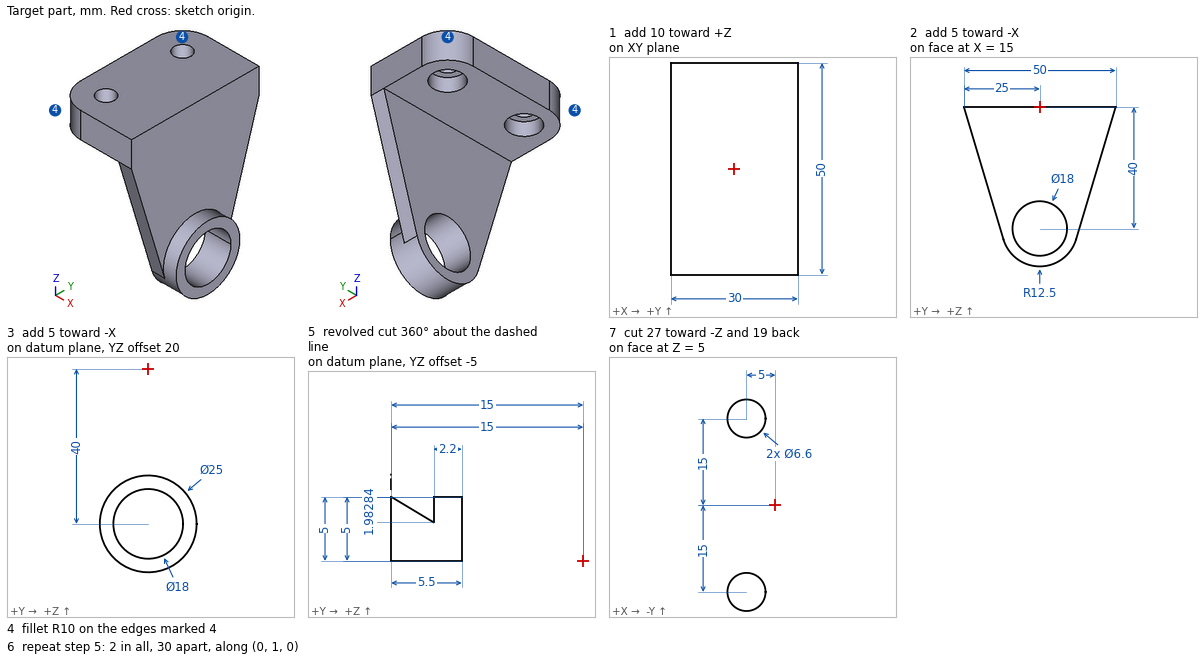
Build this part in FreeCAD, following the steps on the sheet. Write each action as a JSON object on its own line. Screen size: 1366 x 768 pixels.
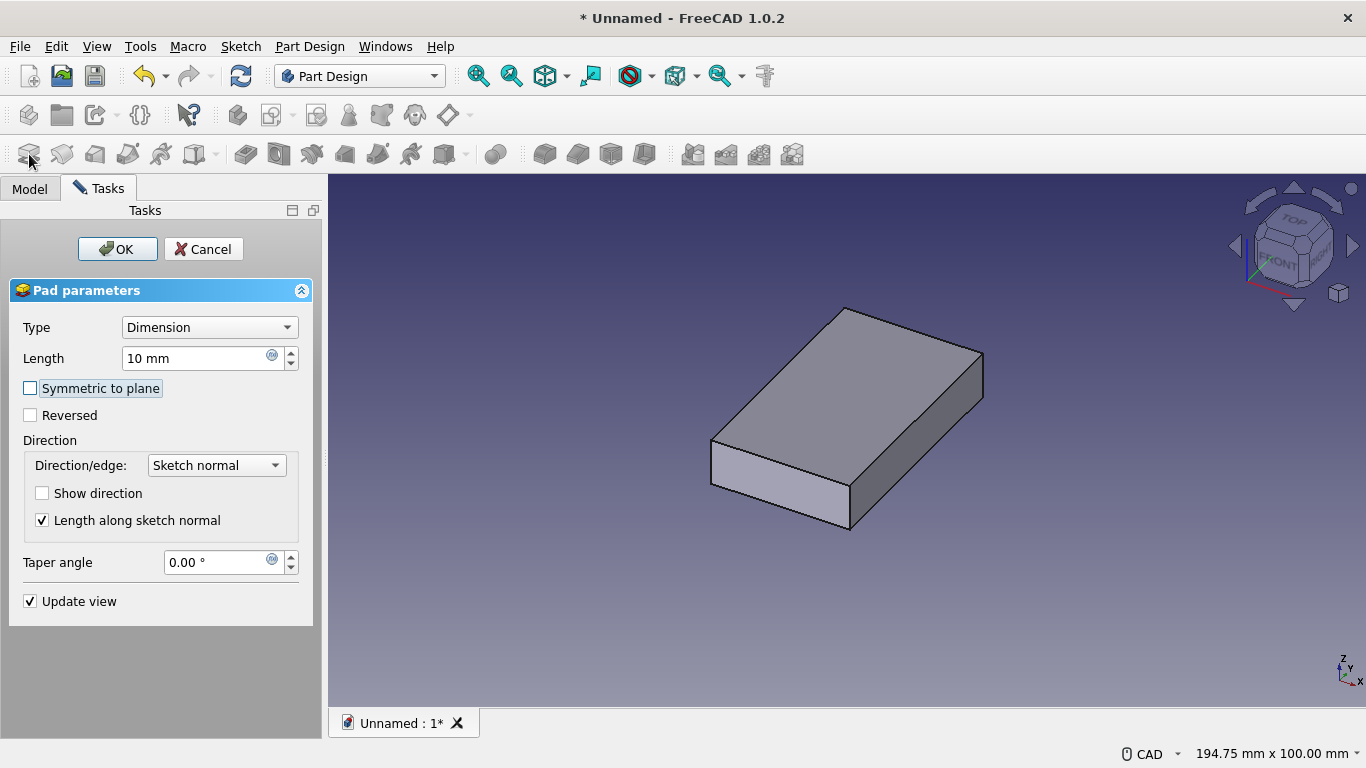
{"action": "left_click", "coordinate": [118, 249]}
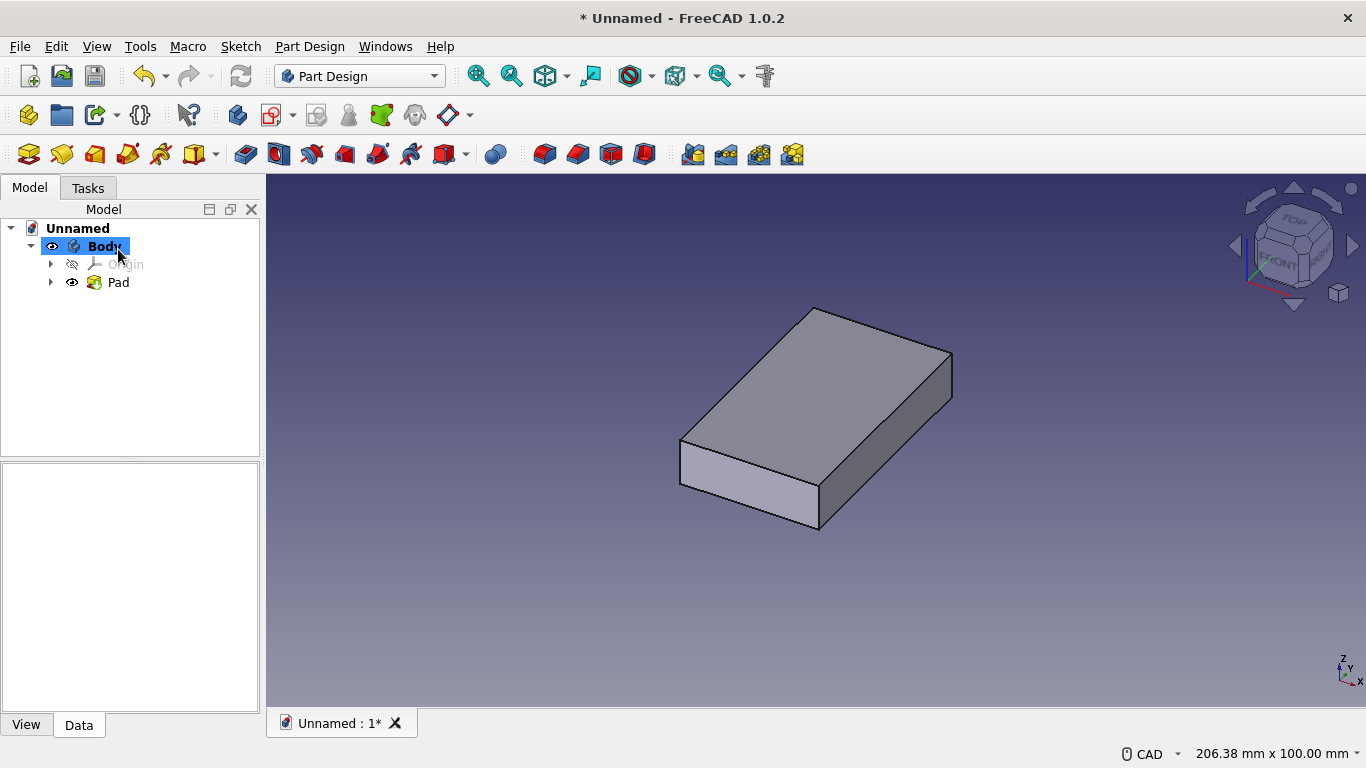
{"action": "key", "text": "v f"}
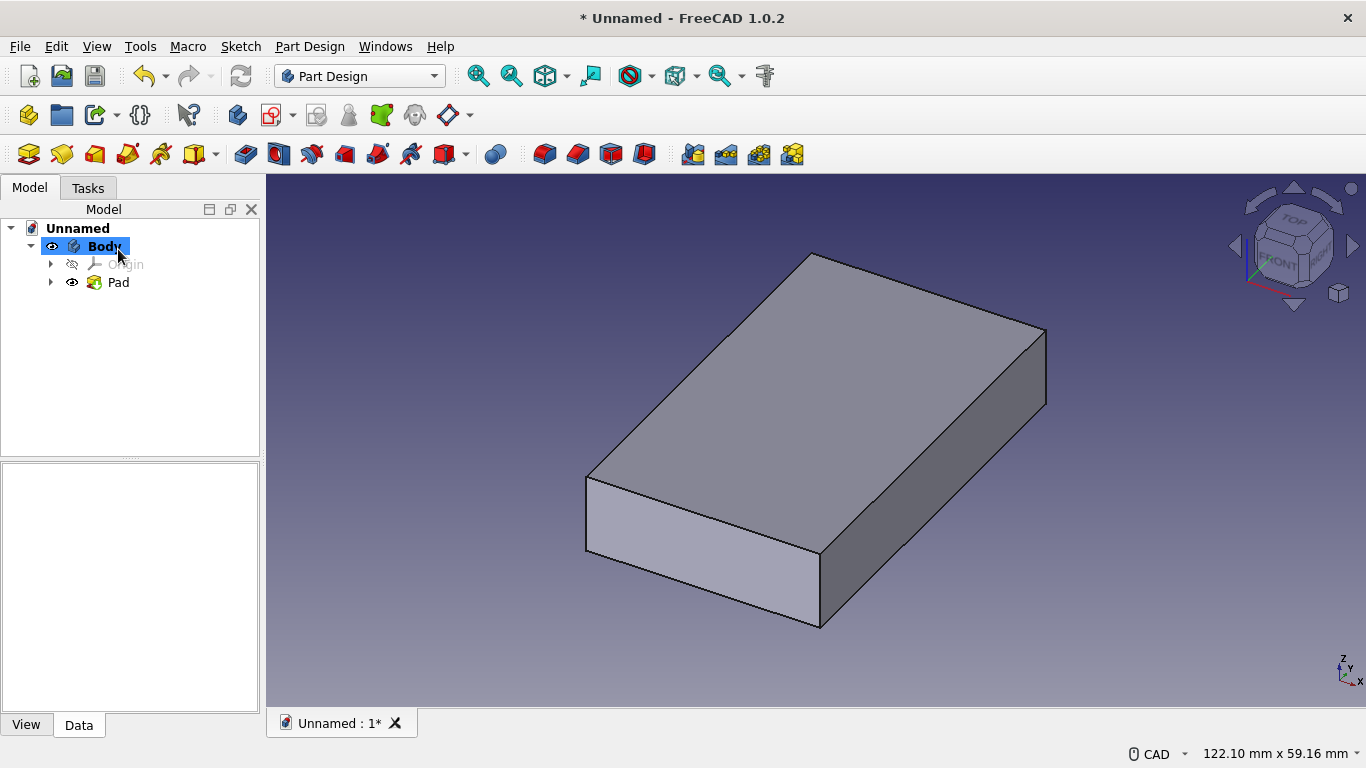
{"action": "left_click", "coordinate": [997, 414]}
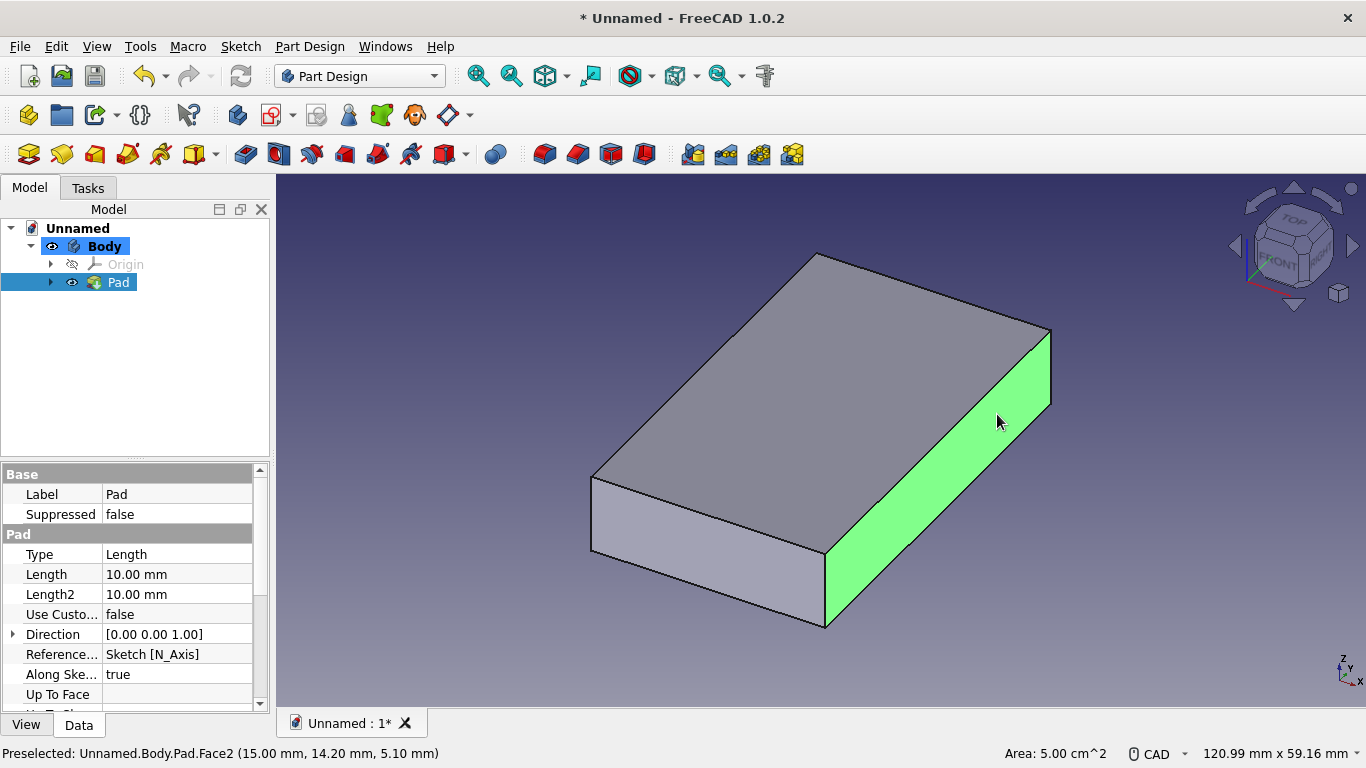
{"action": "left_click", "coordinate": [270, 116]}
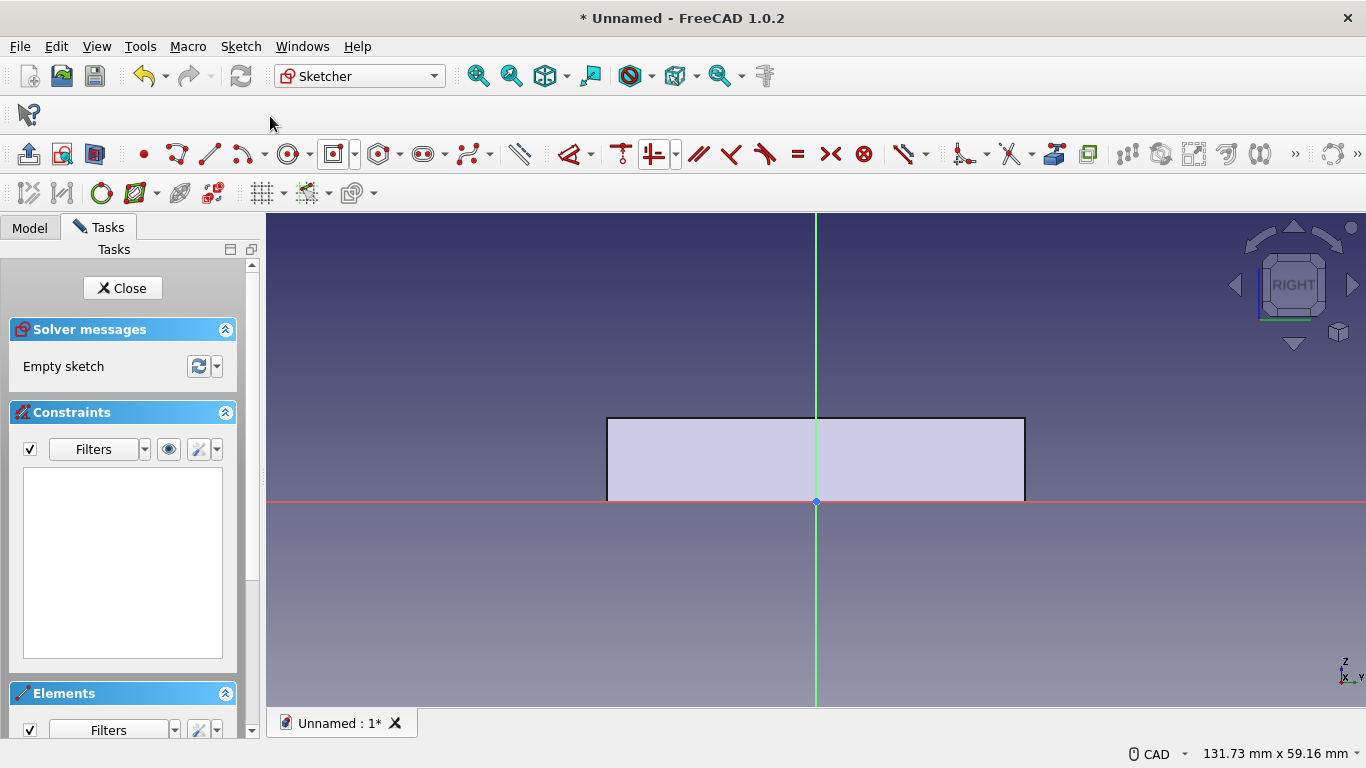
{"action": "scroll", "coordinate": [664, 241], "scroll_direction": "down", "scroll_amount": 3}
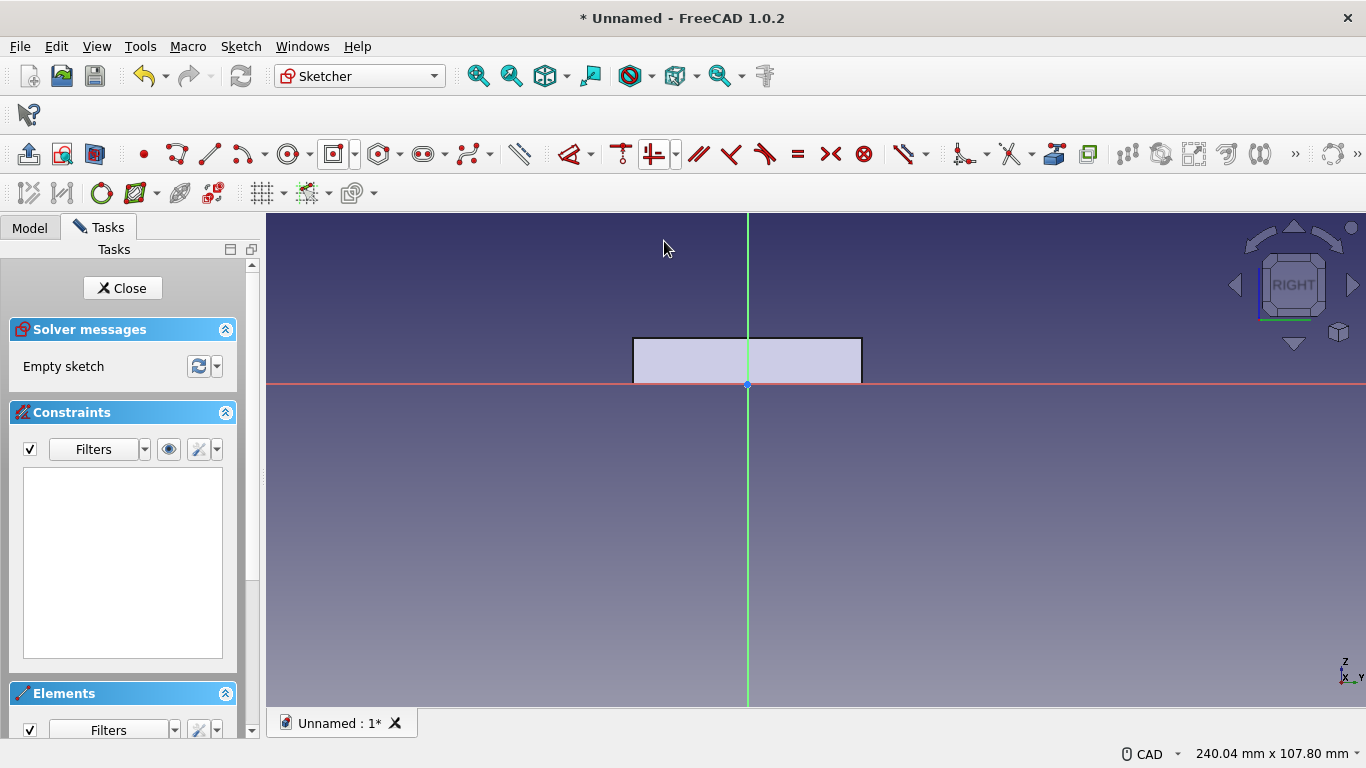
{"action": "left_click", "coordinate": [177, 154]}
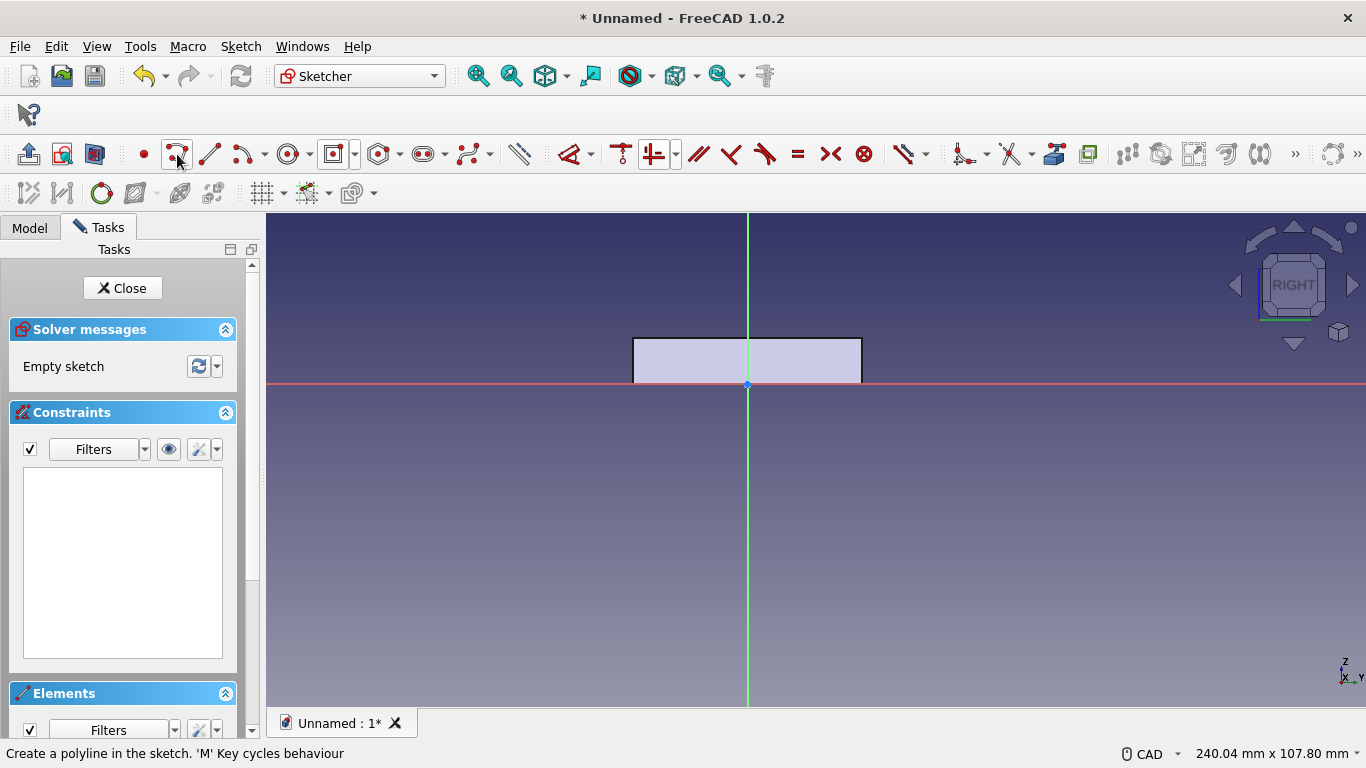
{"action": "left_click", "coordinate": [693, 584]}
{"action": "left_click", "coordinate": [633, 384]}
{"action": "left_click", "coordinate": [862, 393]}
{"action": "left_click", "coordinate": [802, 584]}
{"action": "right_click", "coordinate": [802, 584]}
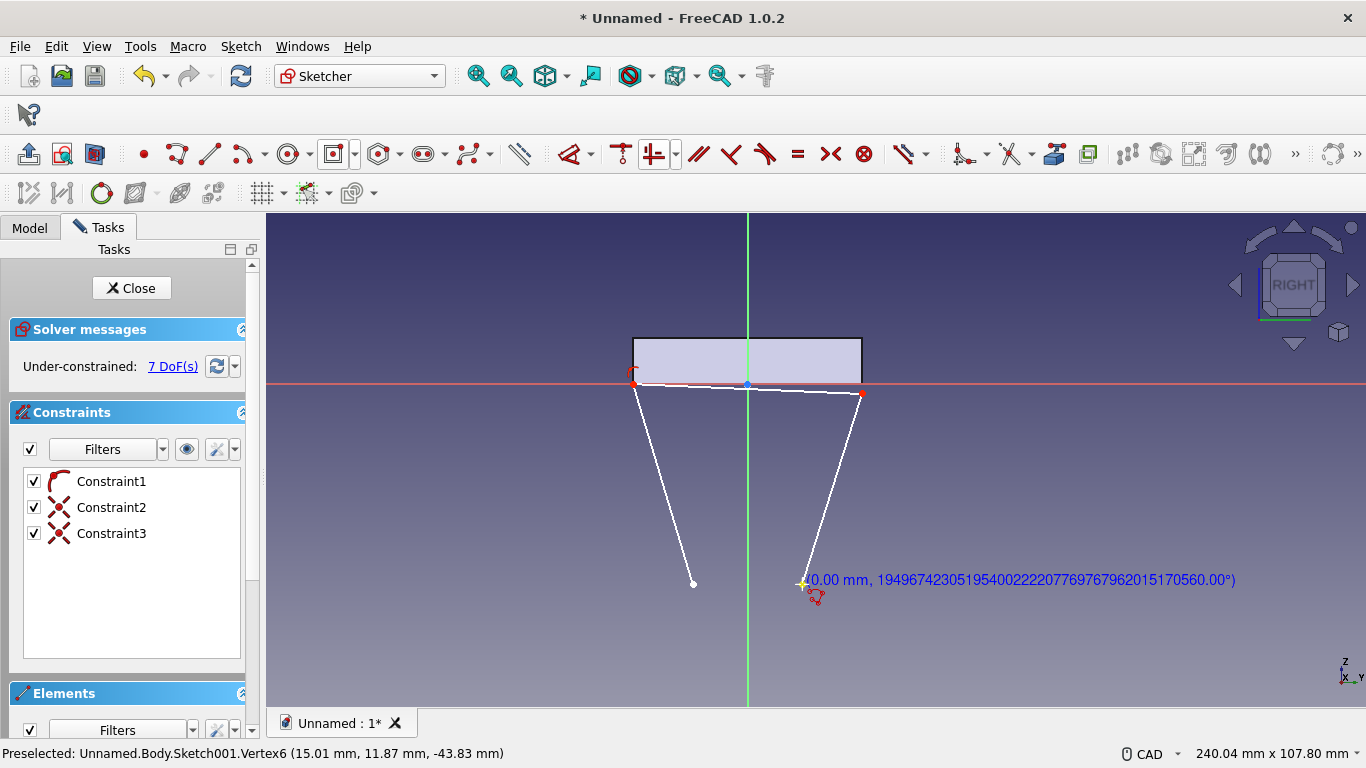
{"action": "key", "text": "g 3 a"}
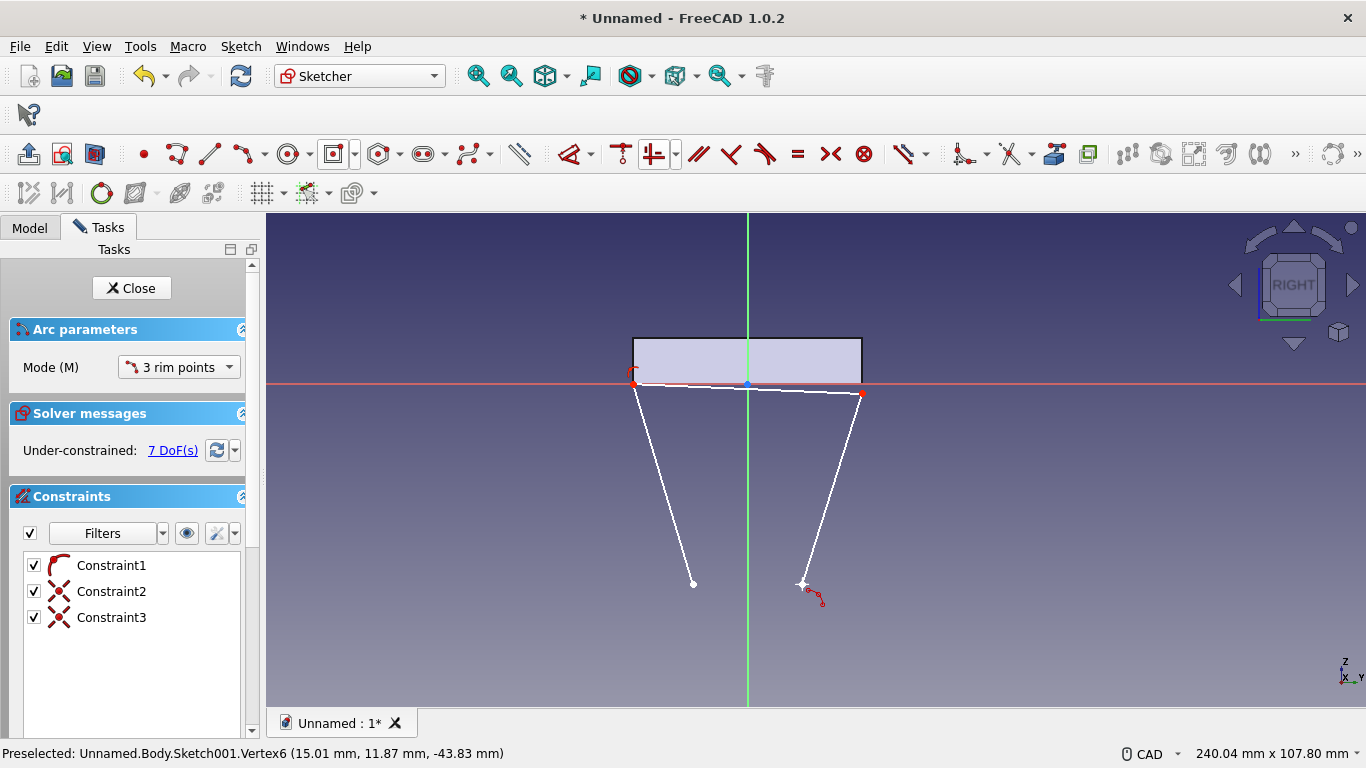
{"action": "left_click", "coordinate": [802, 585]}
{"action": "left_click", "coordinate": [693, 585]}
{"action": "left_click", "coordinate": [733, 623]}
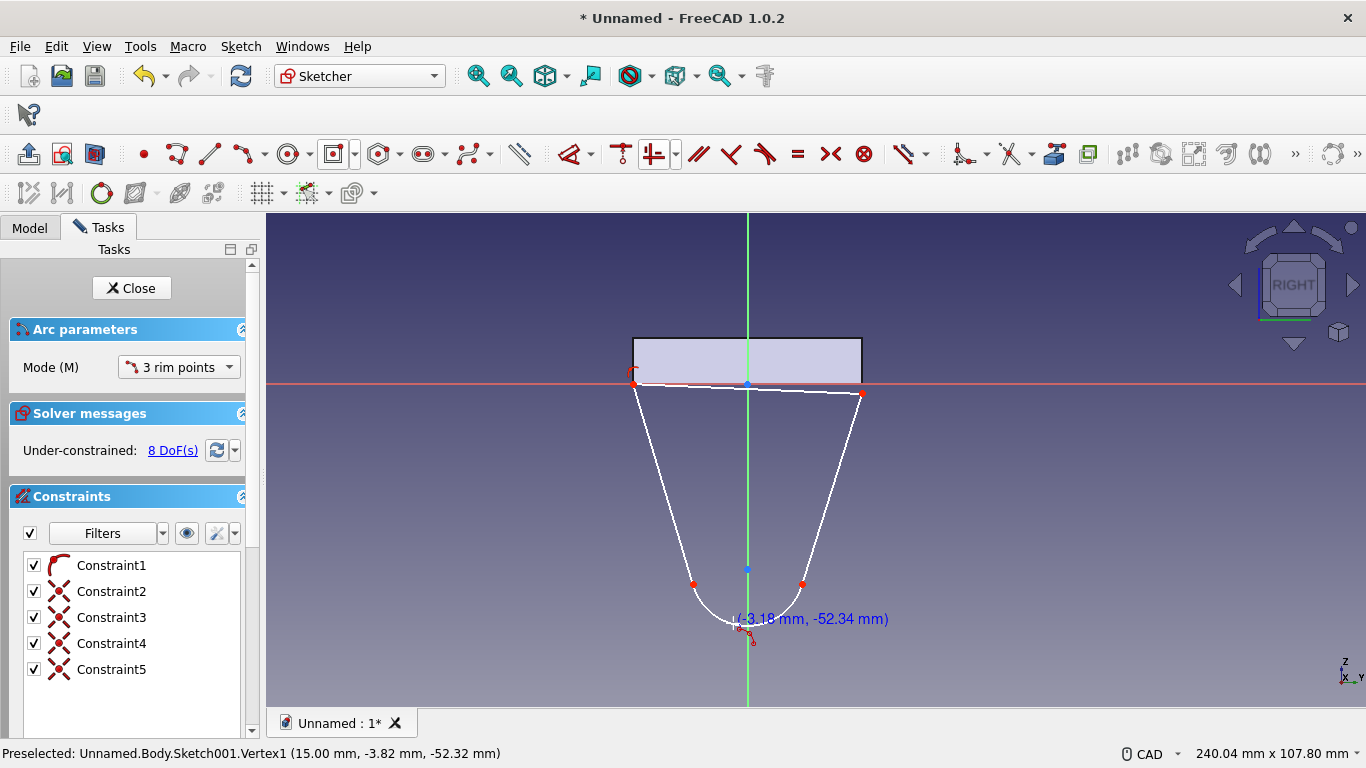
{"action": "key", "text": "g c"}